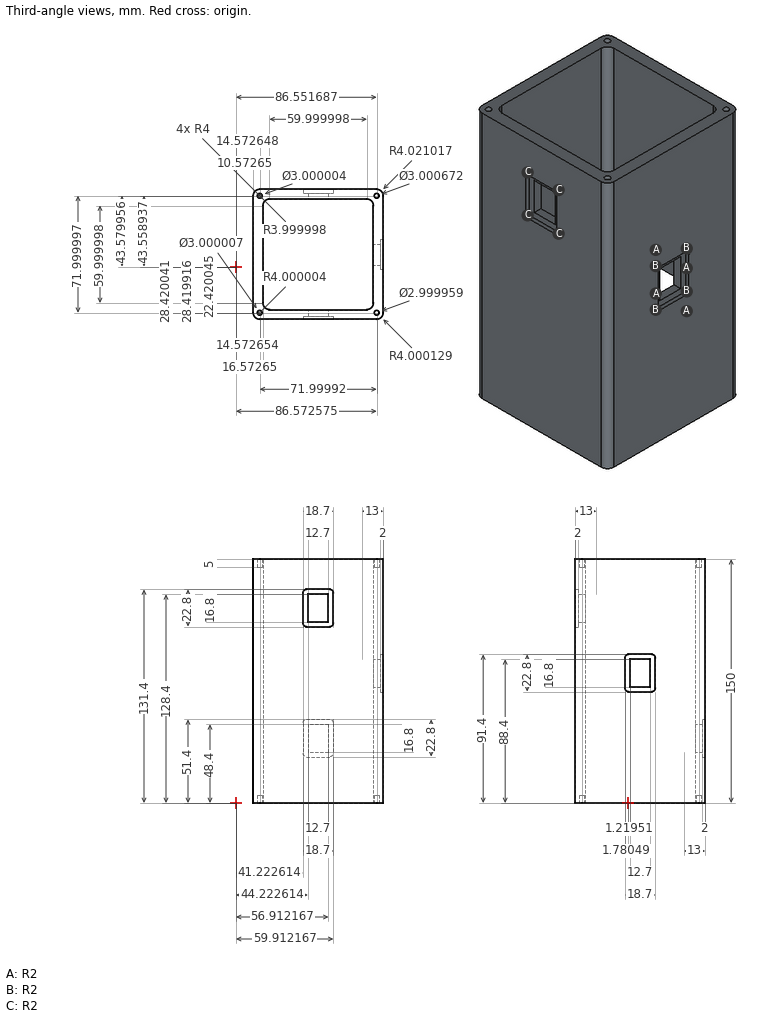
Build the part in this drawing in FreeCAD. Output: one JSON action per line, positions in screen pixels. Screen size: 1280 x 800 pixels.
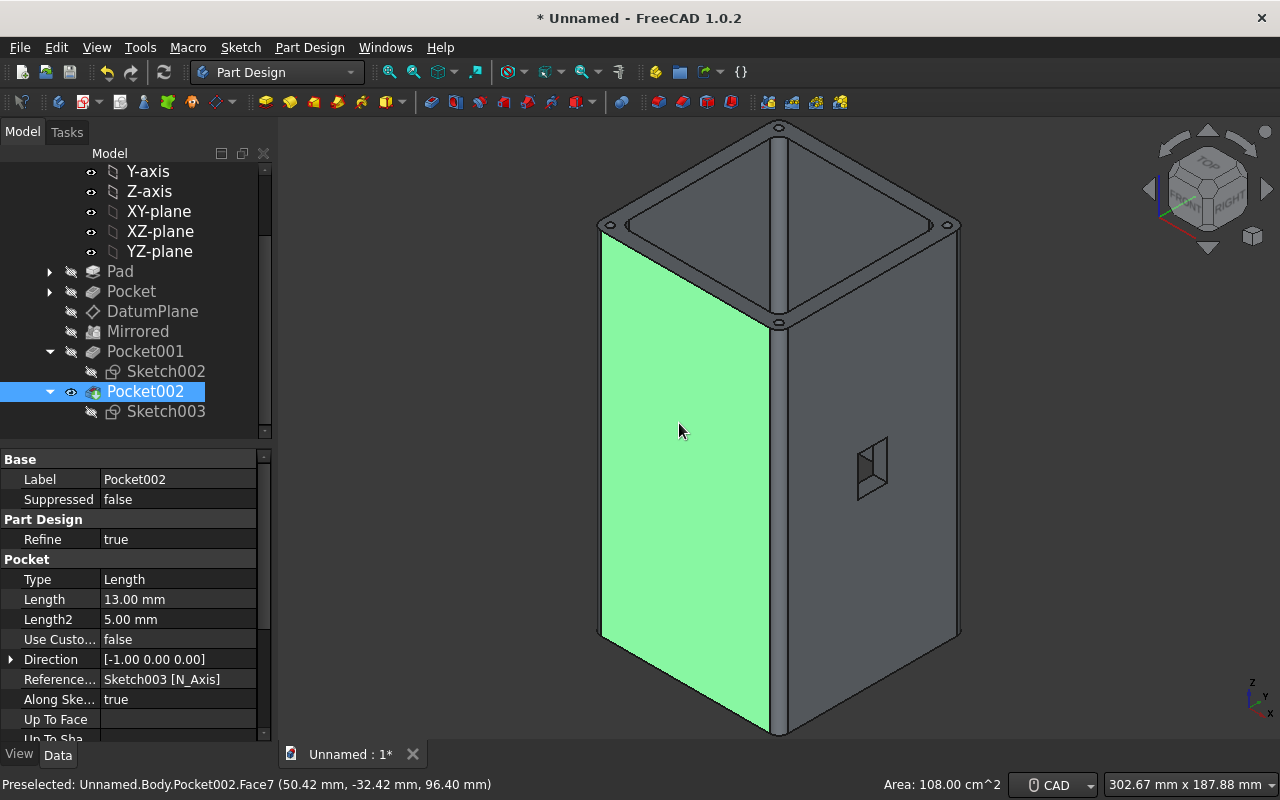
{"action": "left_click", "coordinate": [84, 102]}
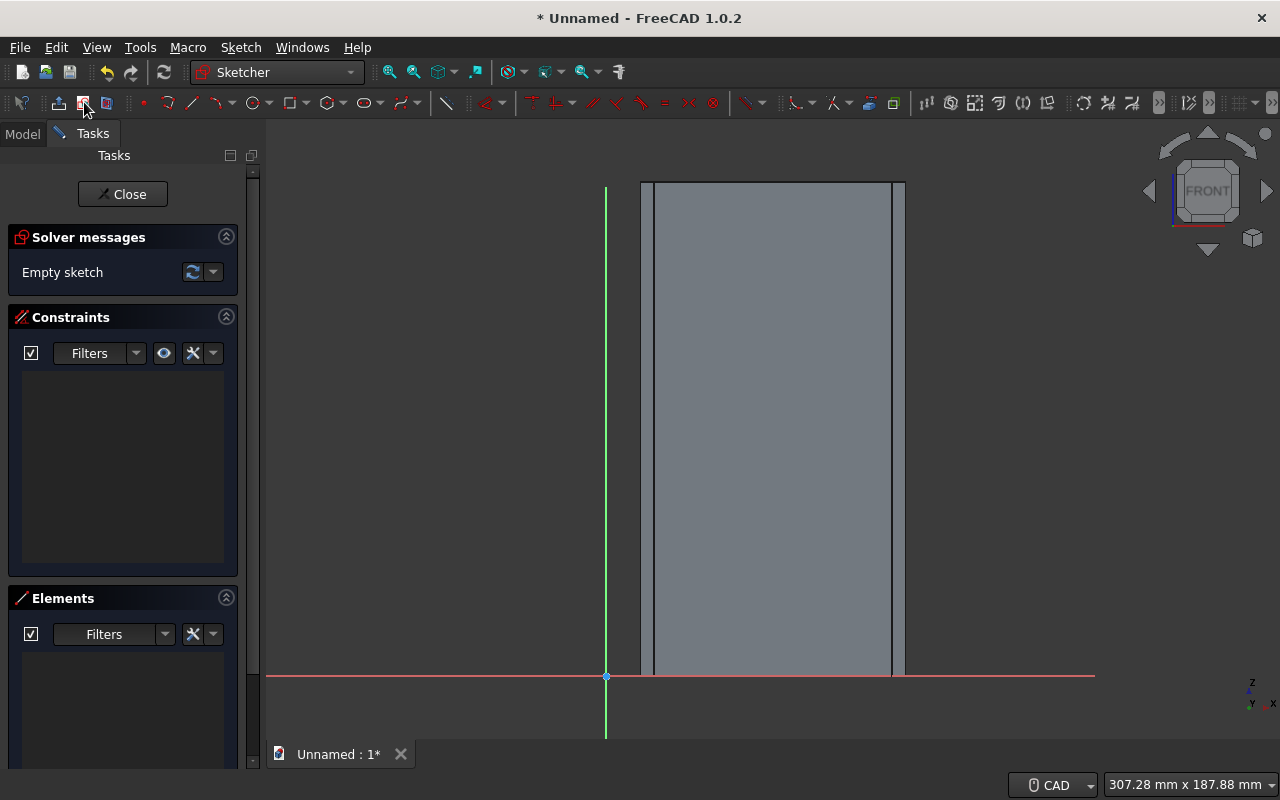
{"action": "scroll", "coordinate": [784, 257], "scroll_direction": "up", "scroll_amount": 10}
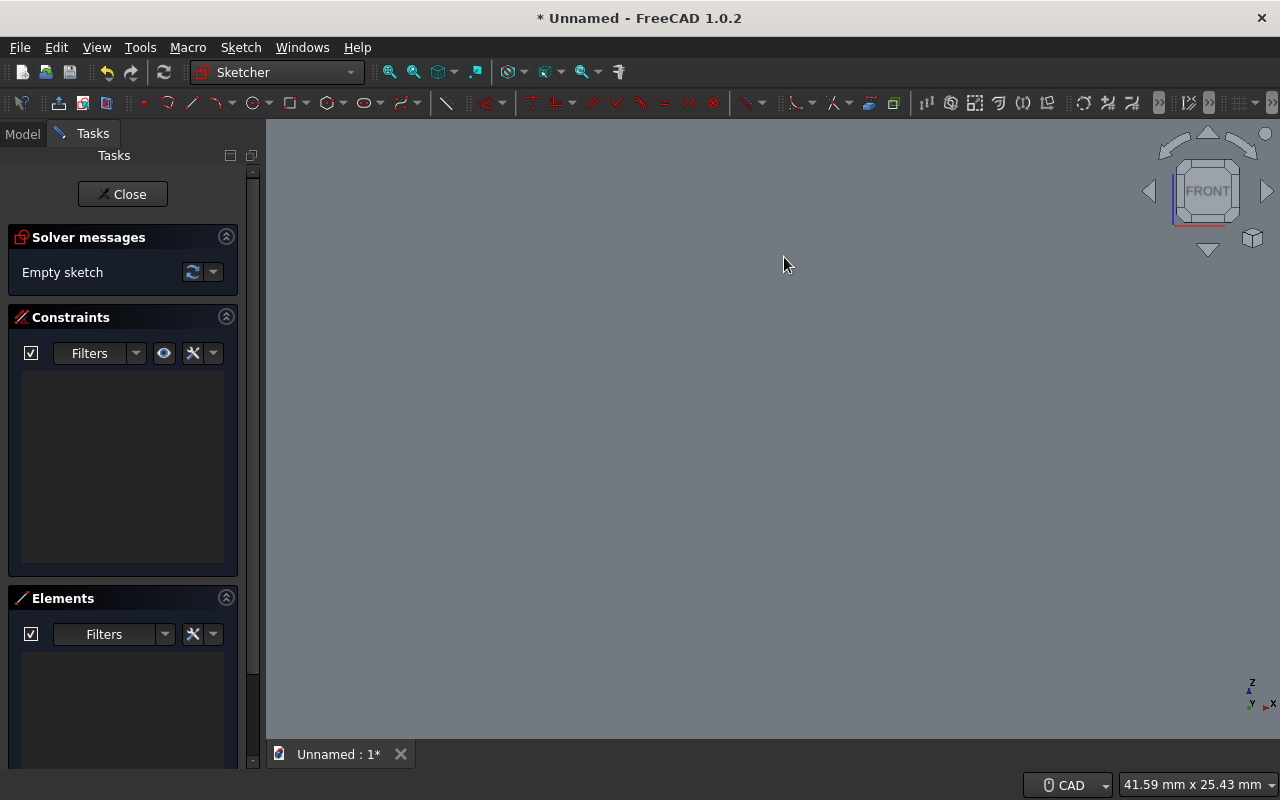
{"action": "left_click", "coordinate": [290, 104]}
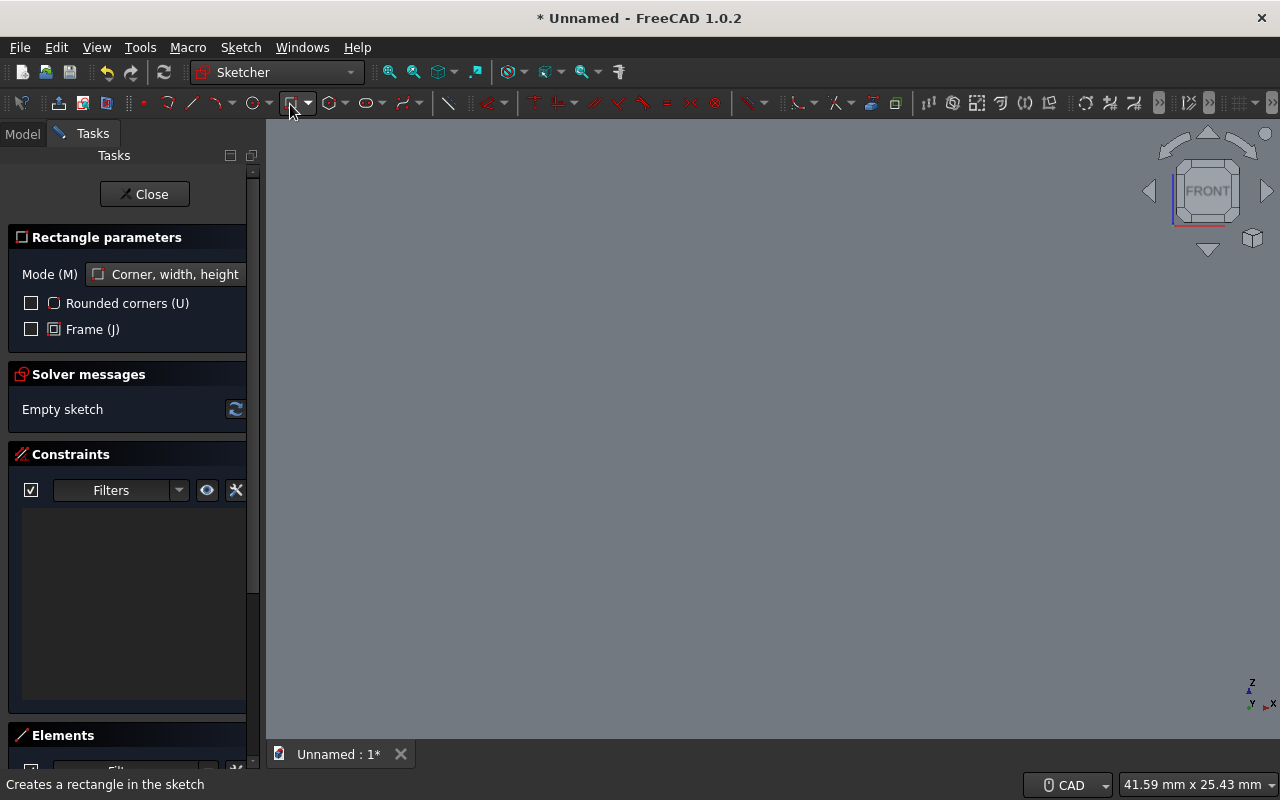
{"action": "left_click", "coordinate": [545, 224]}
{"action": "left_click", "coordinate": [854, 634]}
{"action": "key", "text": "Escape"}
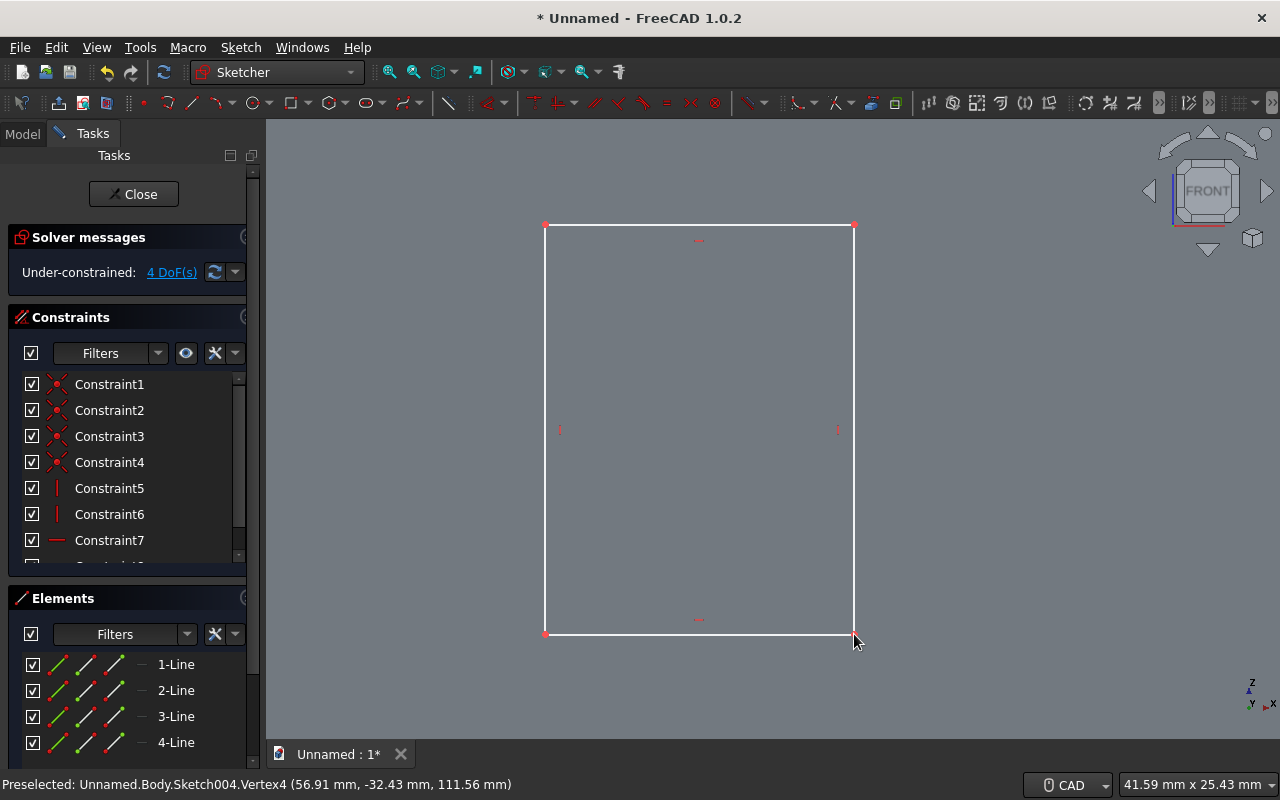
{"action": "left_click", "coordinate": [488, 104]}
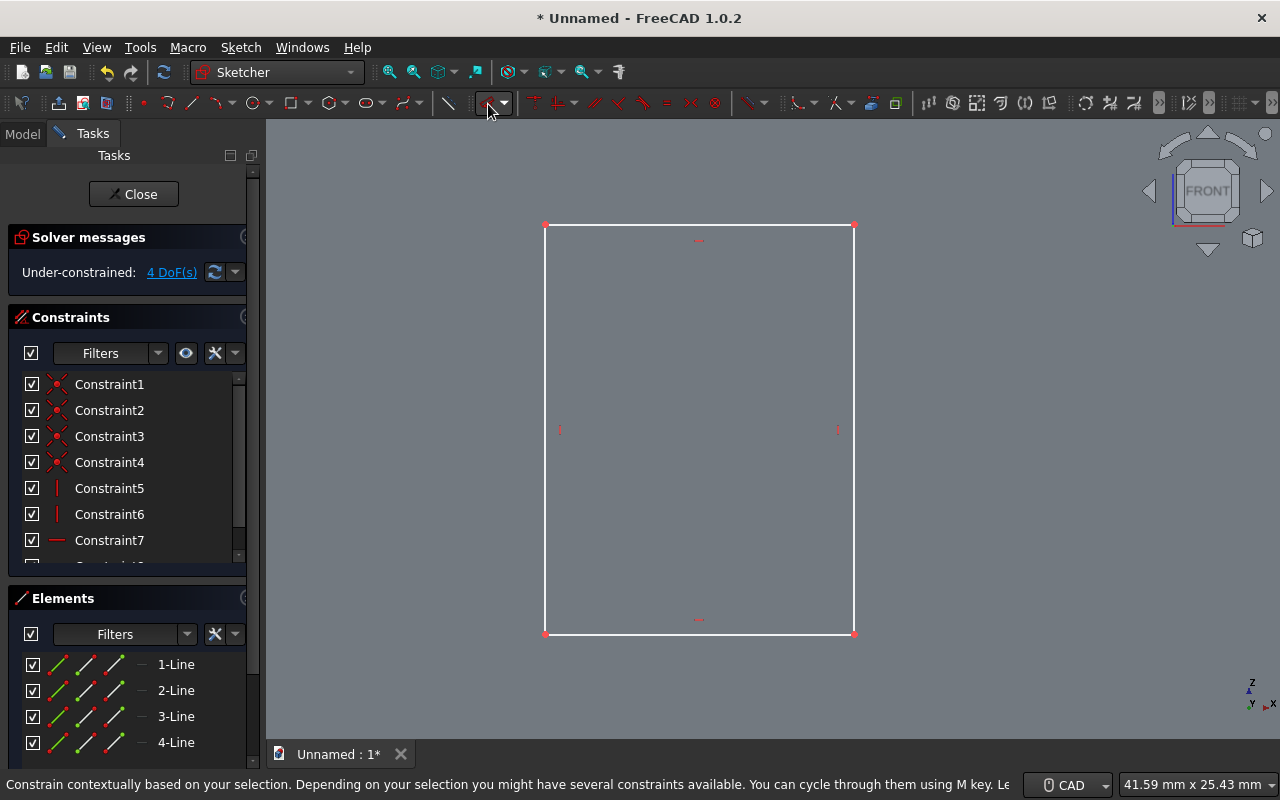
{"action": "left_click", "coordinate": [545, 348]}
{"action": "left_click", "coordinate": [511, 430]}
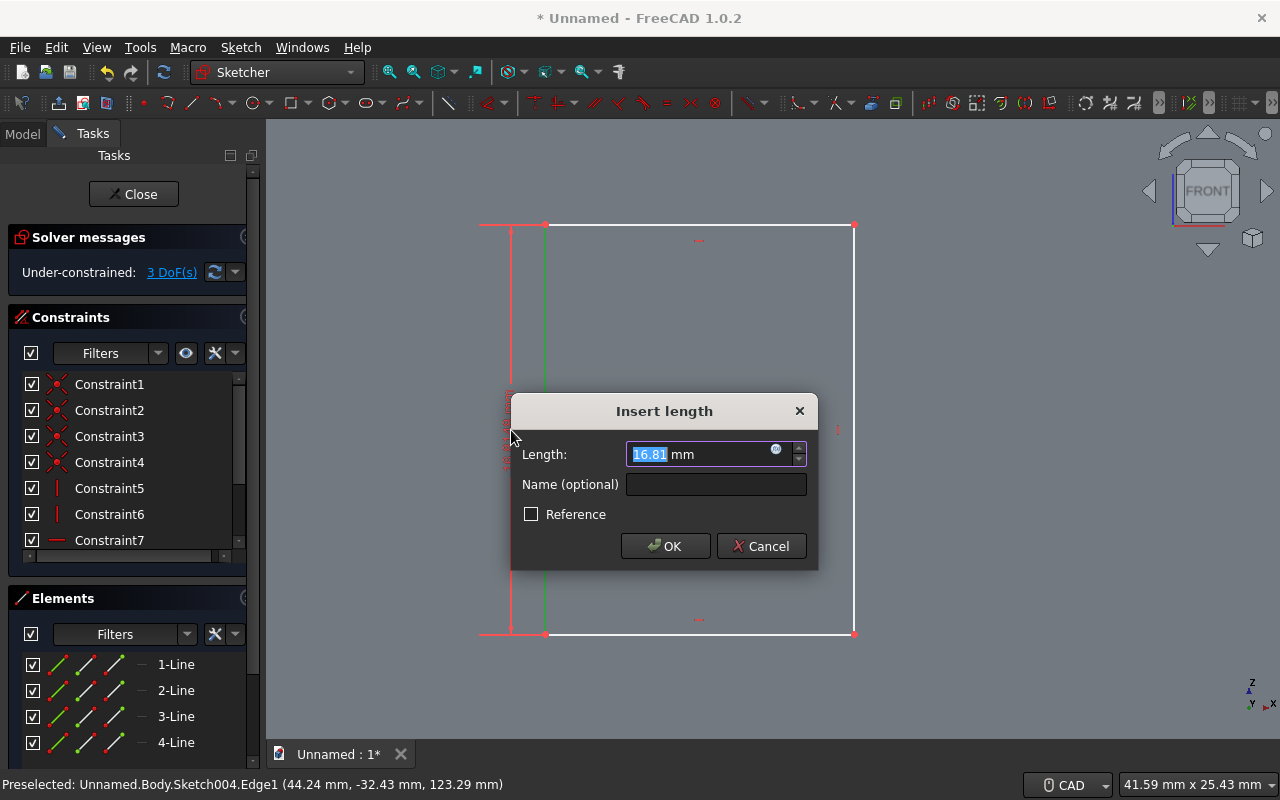
{"action": "type", "text": "16.8"}
{"action": "key", "text": "Return"}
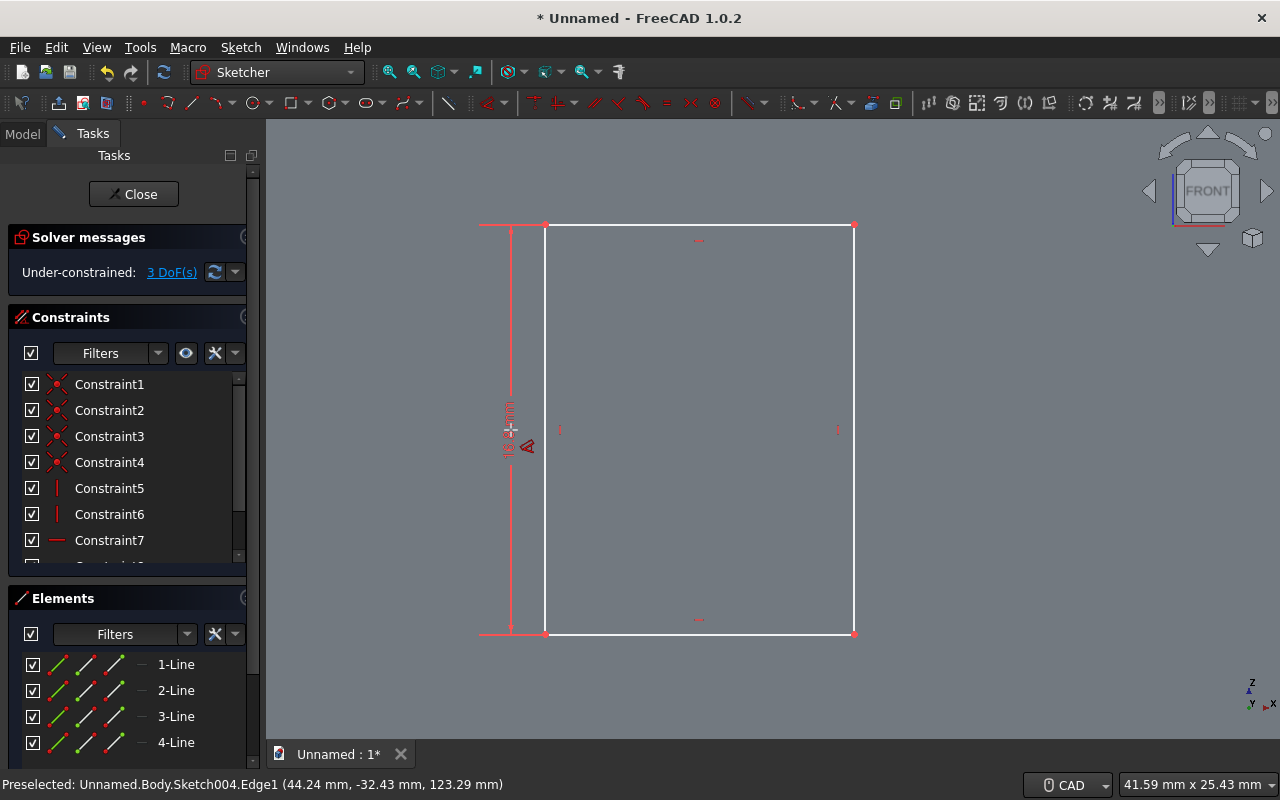
{"action": "left_click", "coordinate": [638, 635]}
{"action": "left_click", "coordinate": [700, 669]}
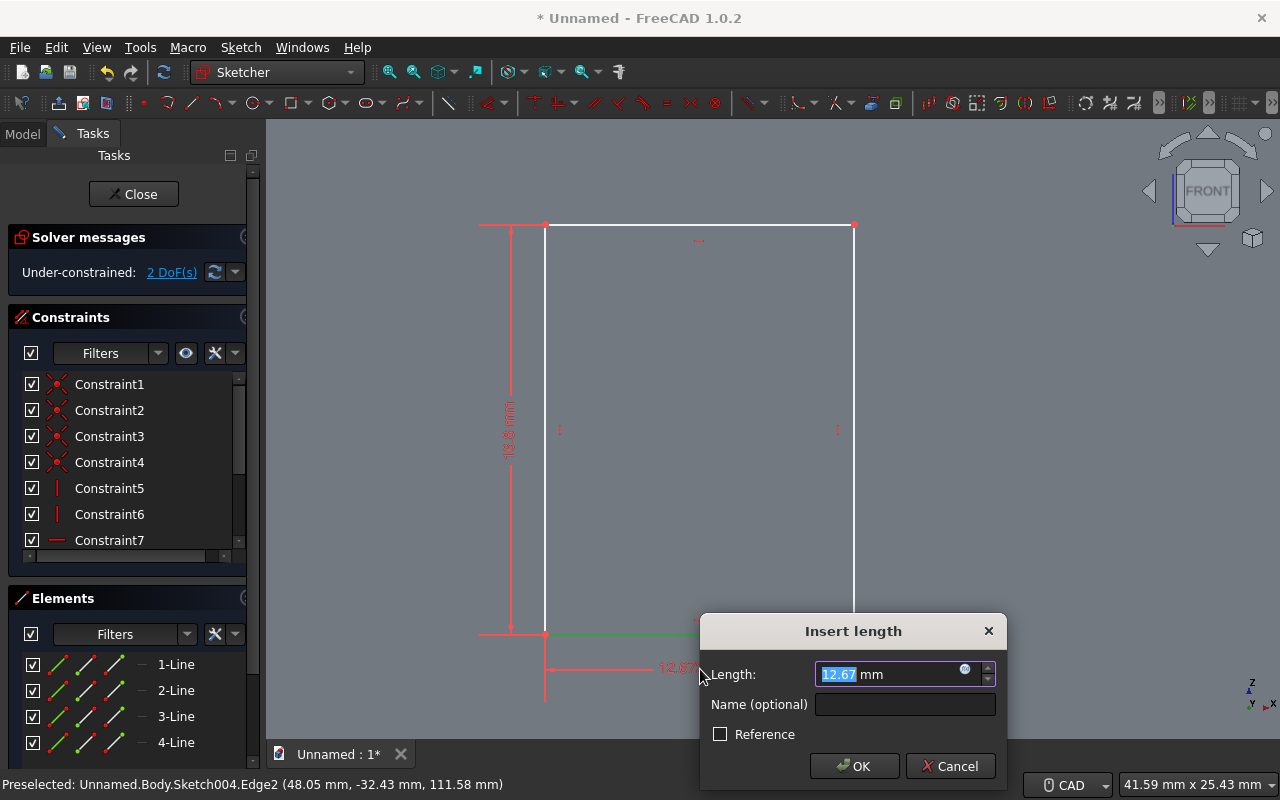
{"action": "type", "text": "12.7"}
{"action": "key", "text": "Return"}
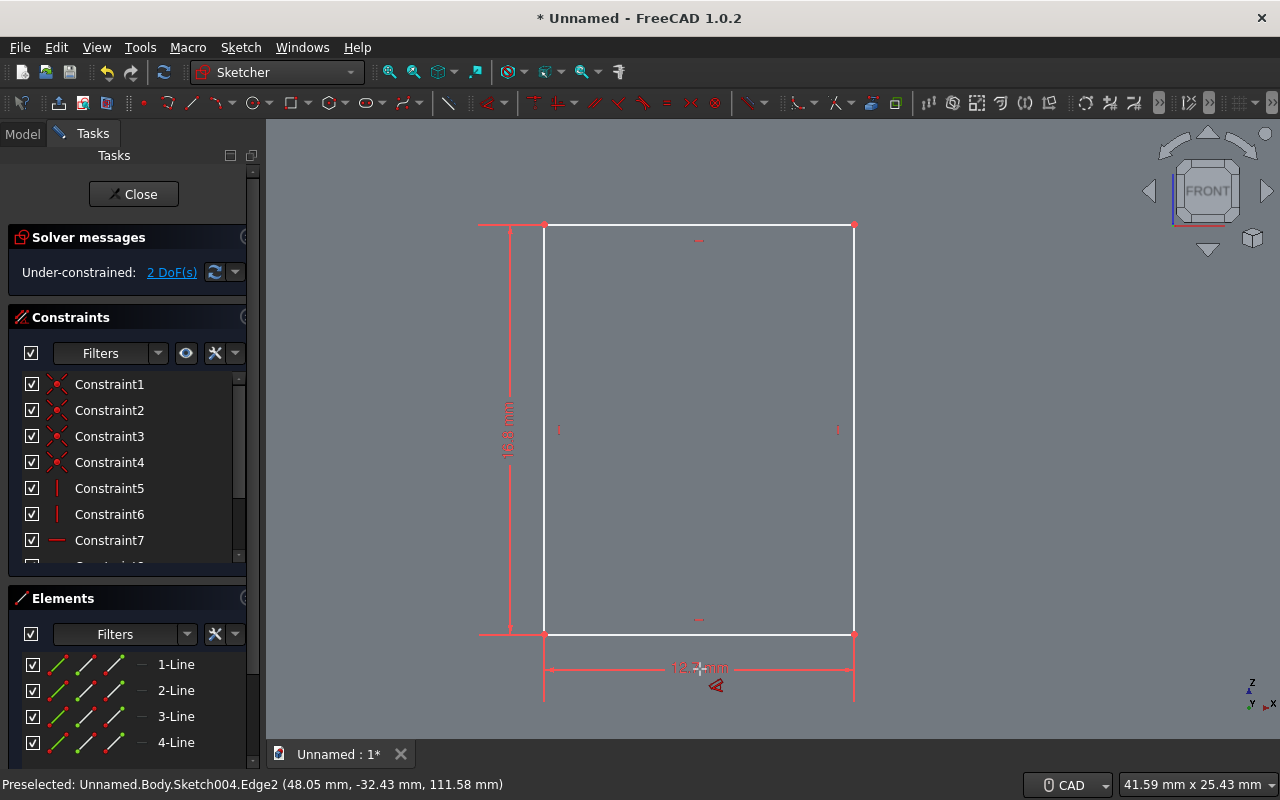
{"action": "left_click", "coordinate": [544, 225]}
{"action": "left_click", "coordinate": [578, 468]}